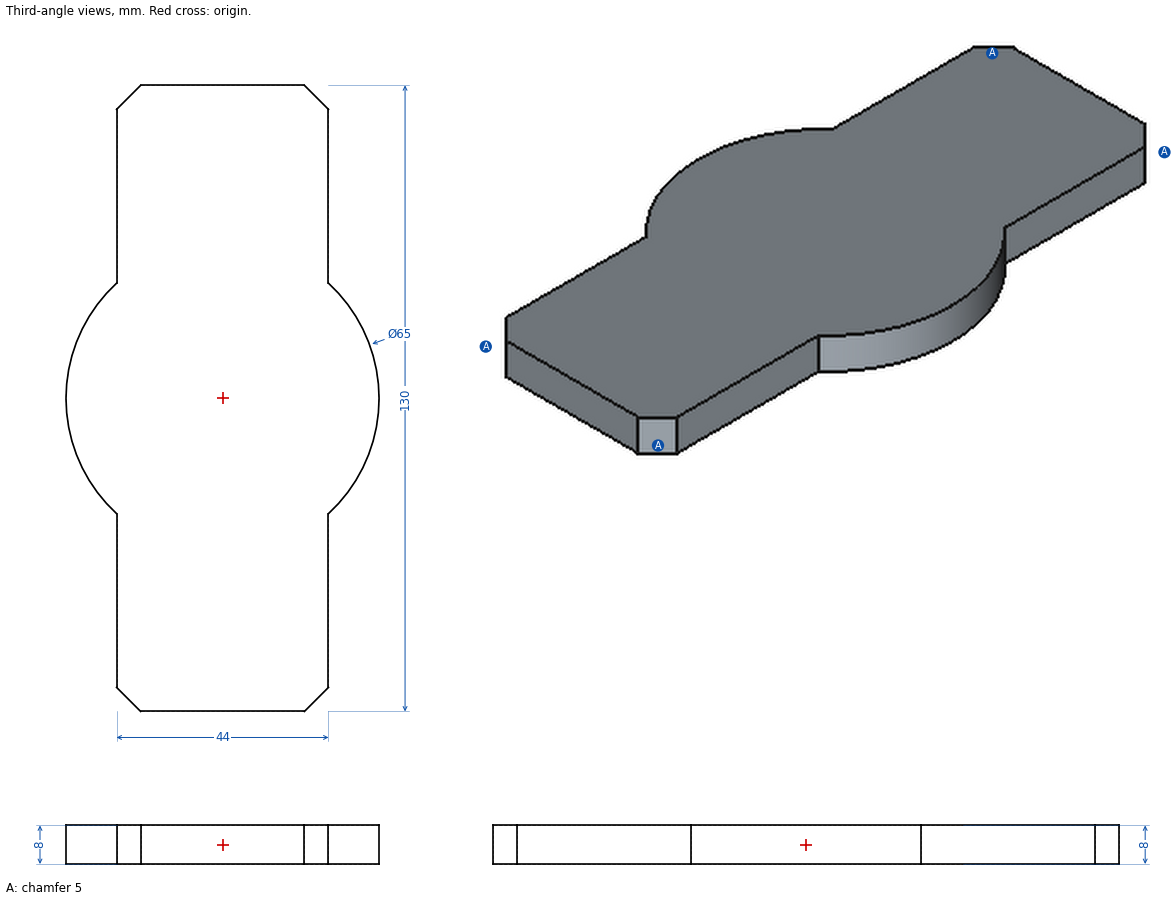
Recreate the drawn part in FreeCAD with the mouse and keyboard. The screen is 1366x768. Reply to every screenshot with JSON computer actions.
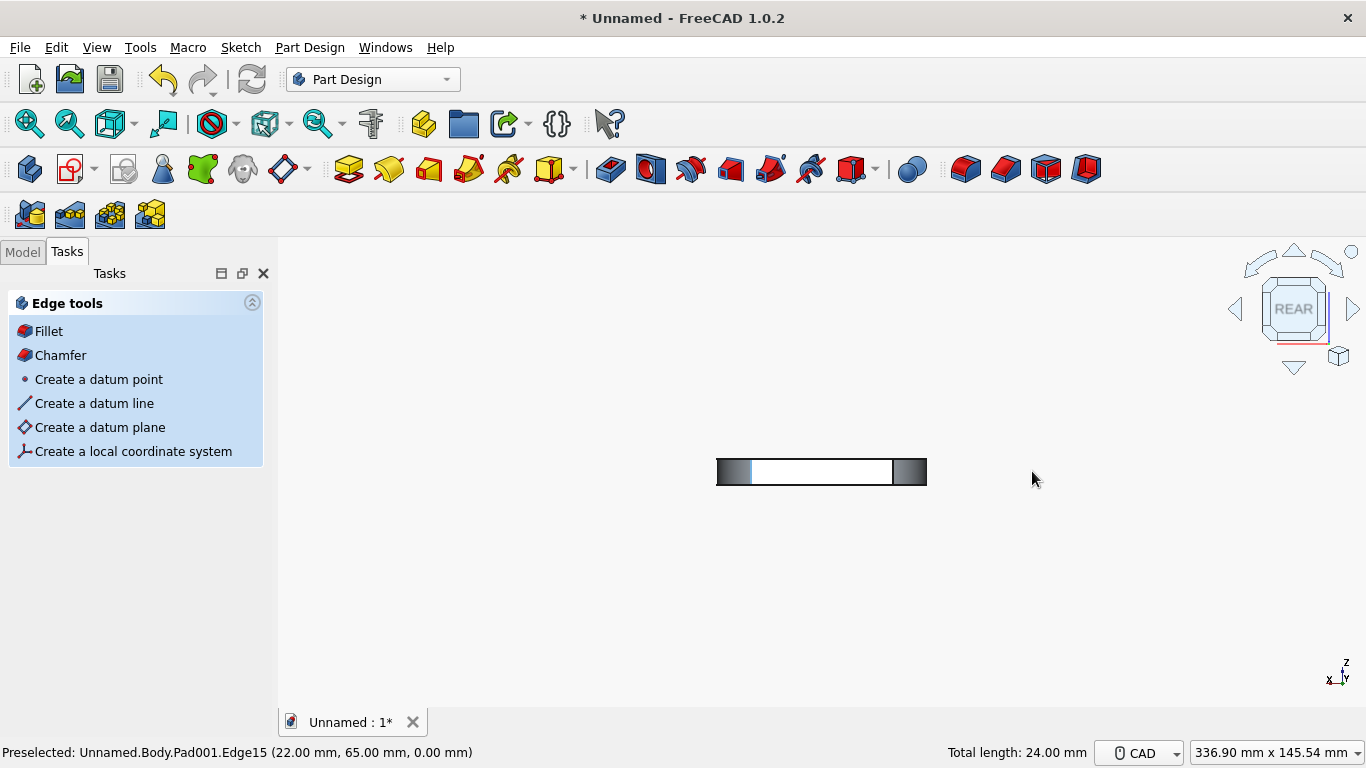
{"action": "left_click", "coordinate": [30, 124]}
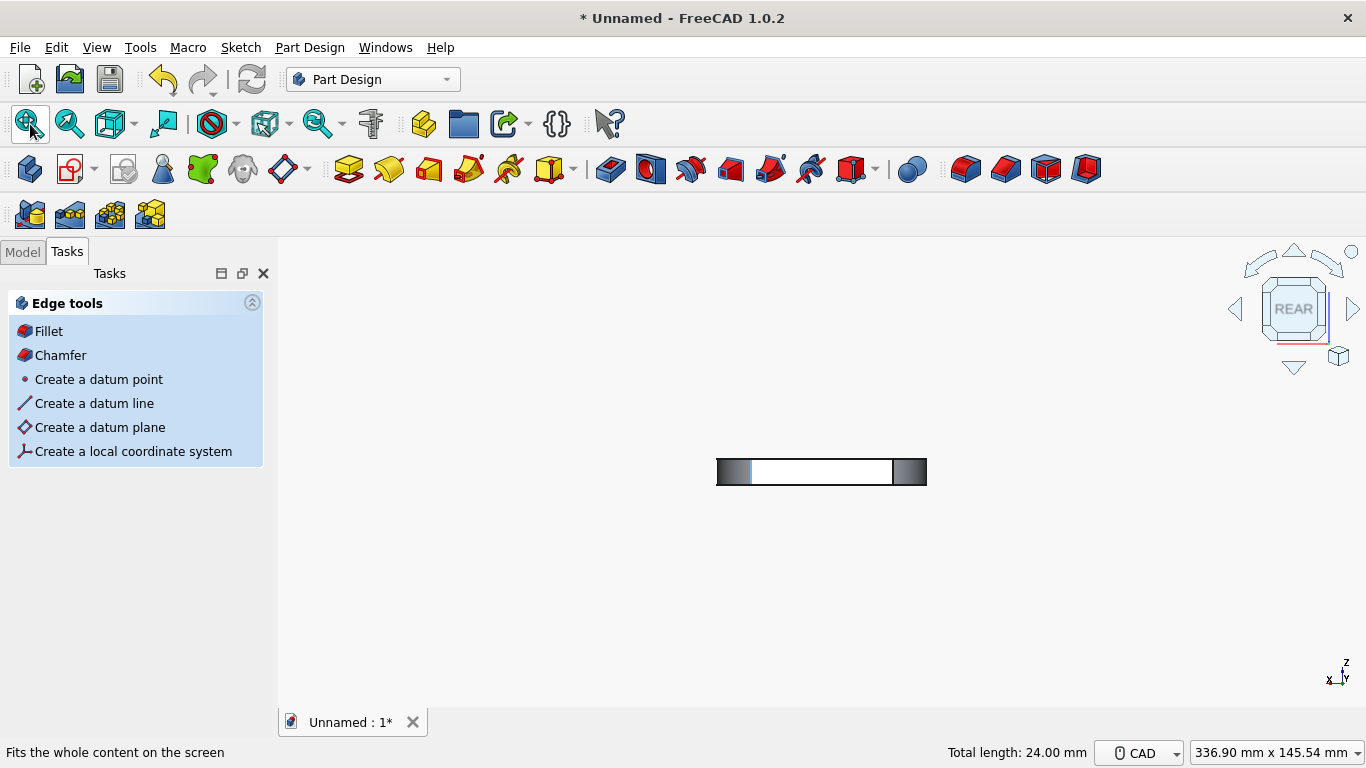
{"action": "left_click", "coordinate": [893, 471], "text": "ctrl"}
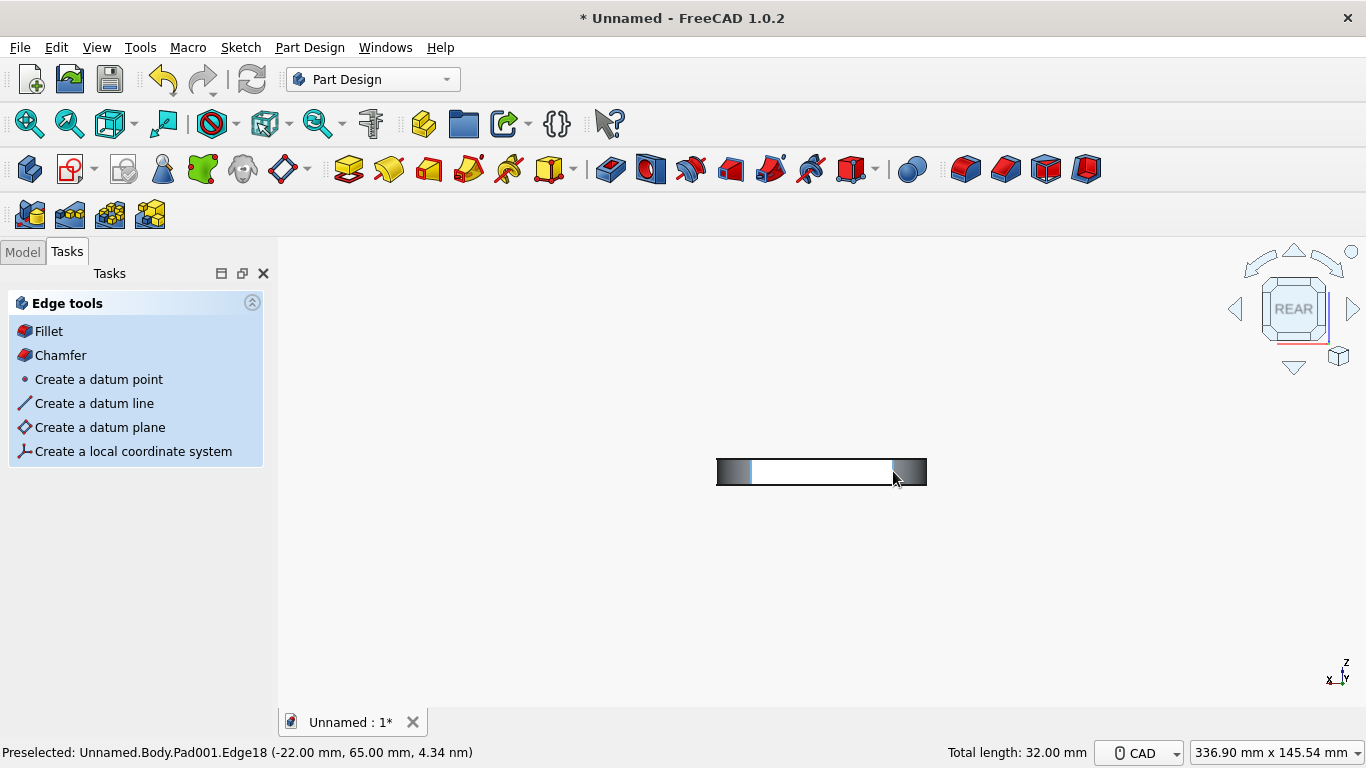
{"action": "left_click", "coordinate": [1006, 170]}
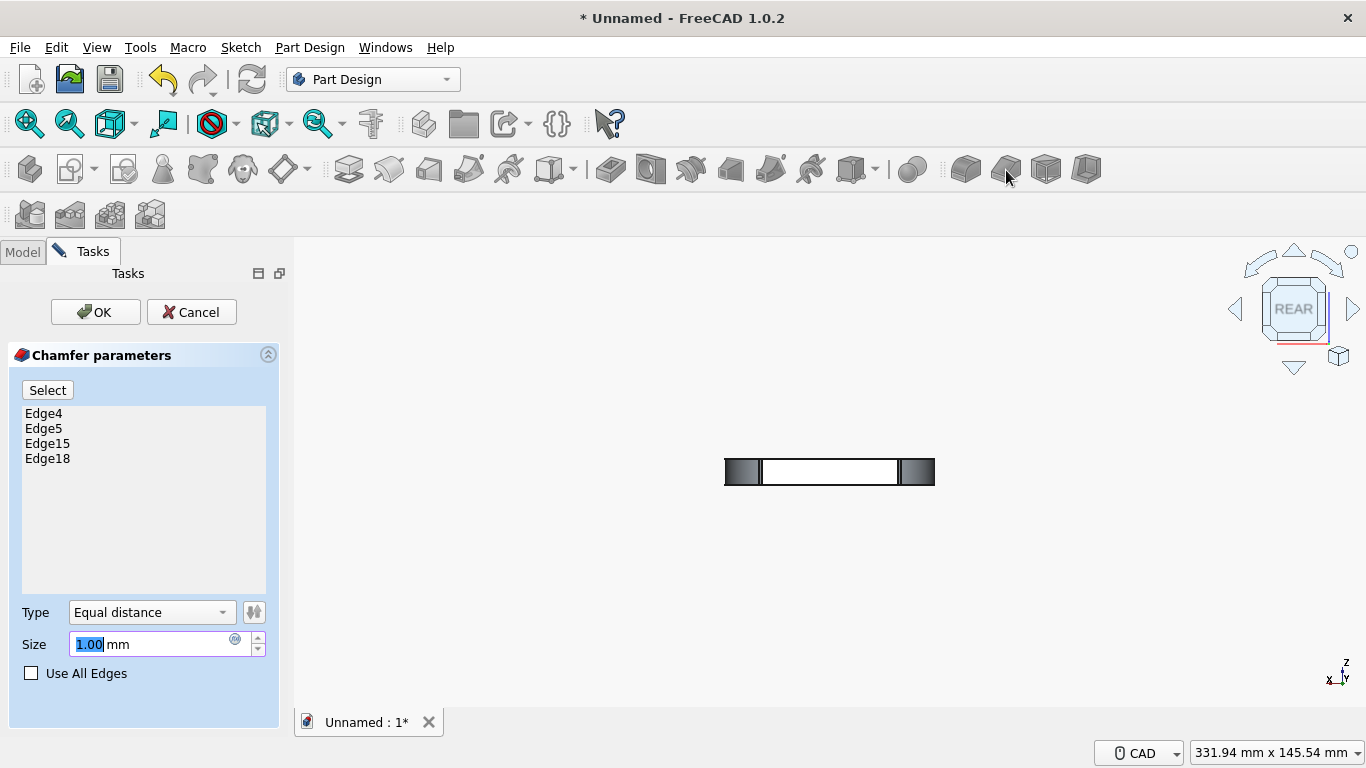
{"action": "type", "text": "5"}
{"action": "key", "text": "Tab"}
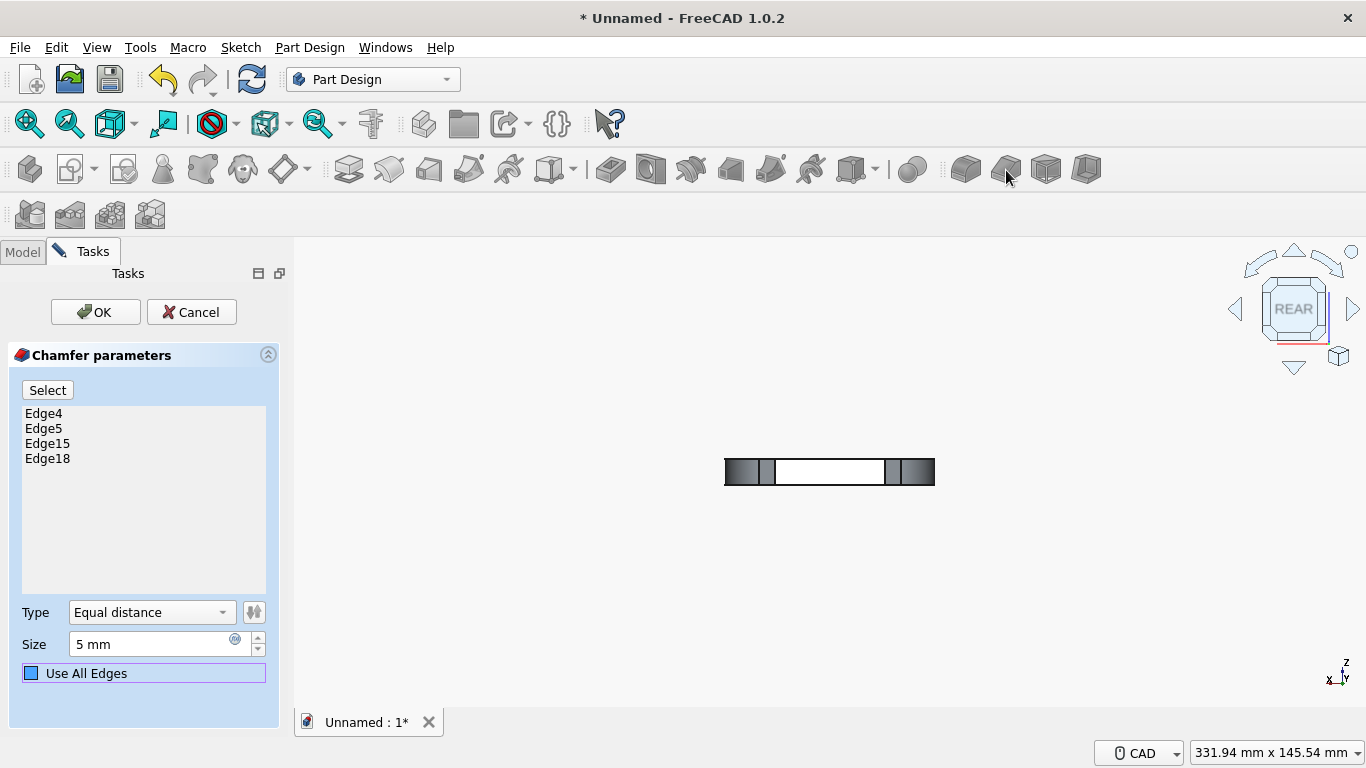
{"action": "left_click", "coordinate": [96, 312]}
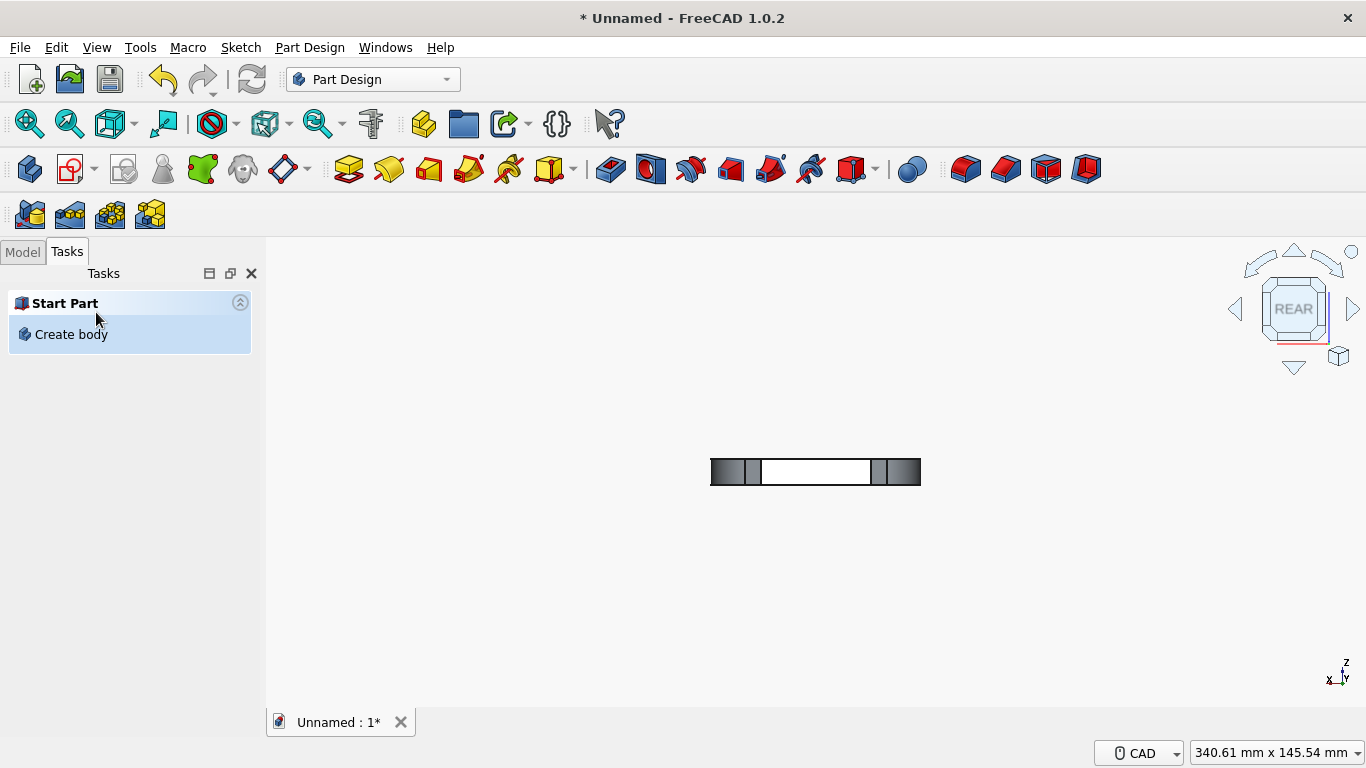
{"action": "key", "text": "0"}